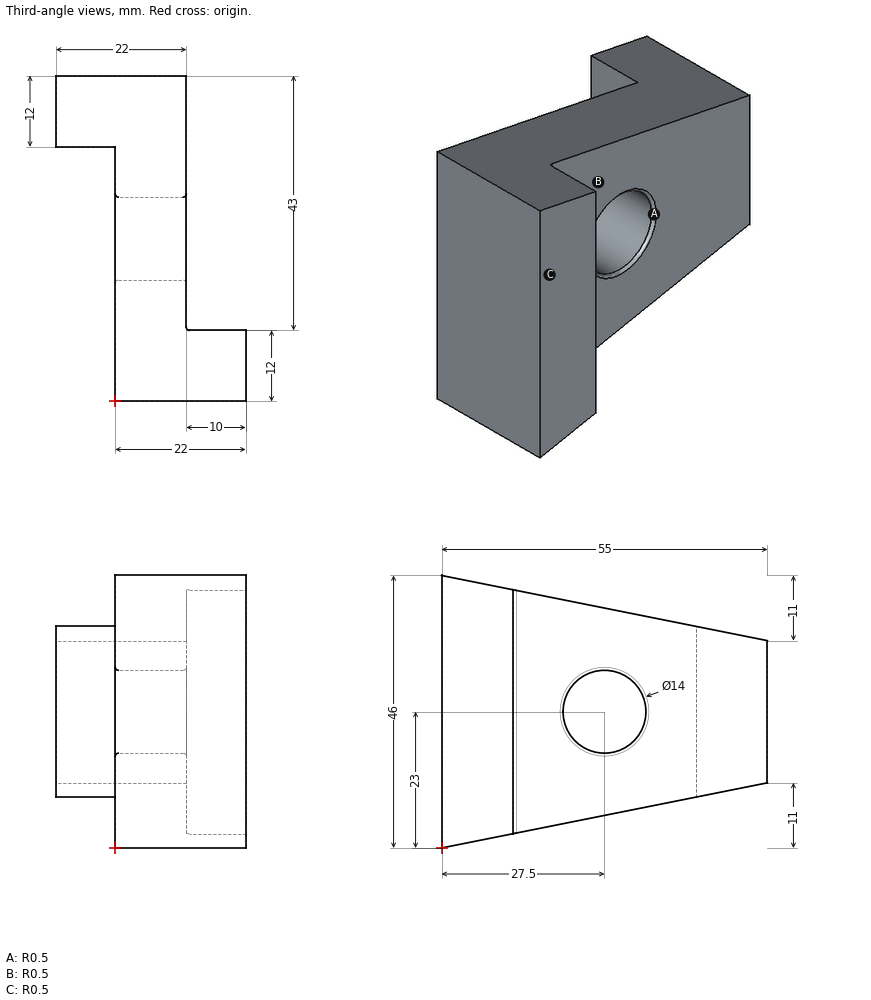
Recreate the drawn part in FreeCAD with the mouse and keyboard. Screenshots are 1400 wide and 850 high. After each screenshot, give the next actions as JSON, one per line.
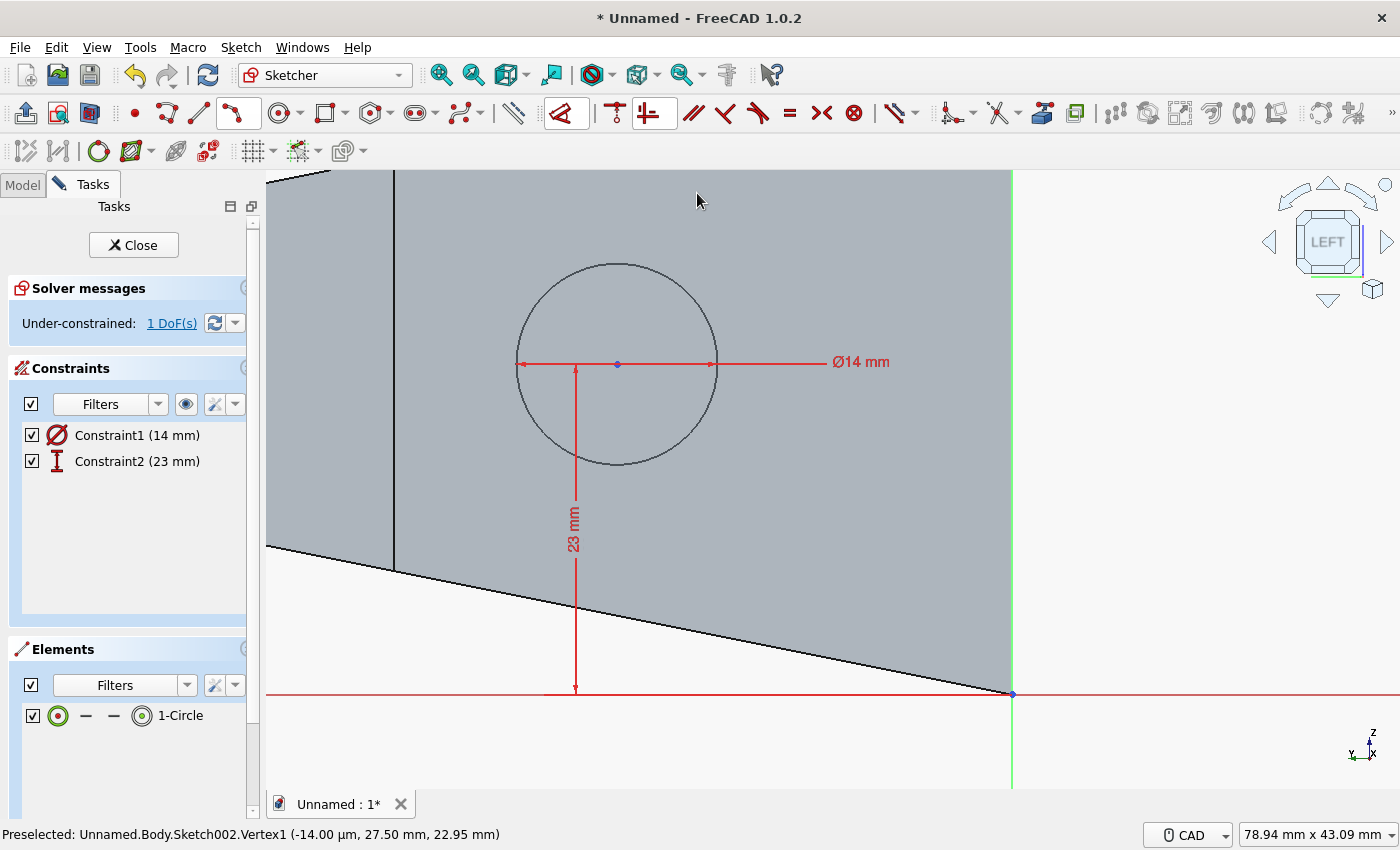
{"action": "left_click", "coordinate": [617, 364]}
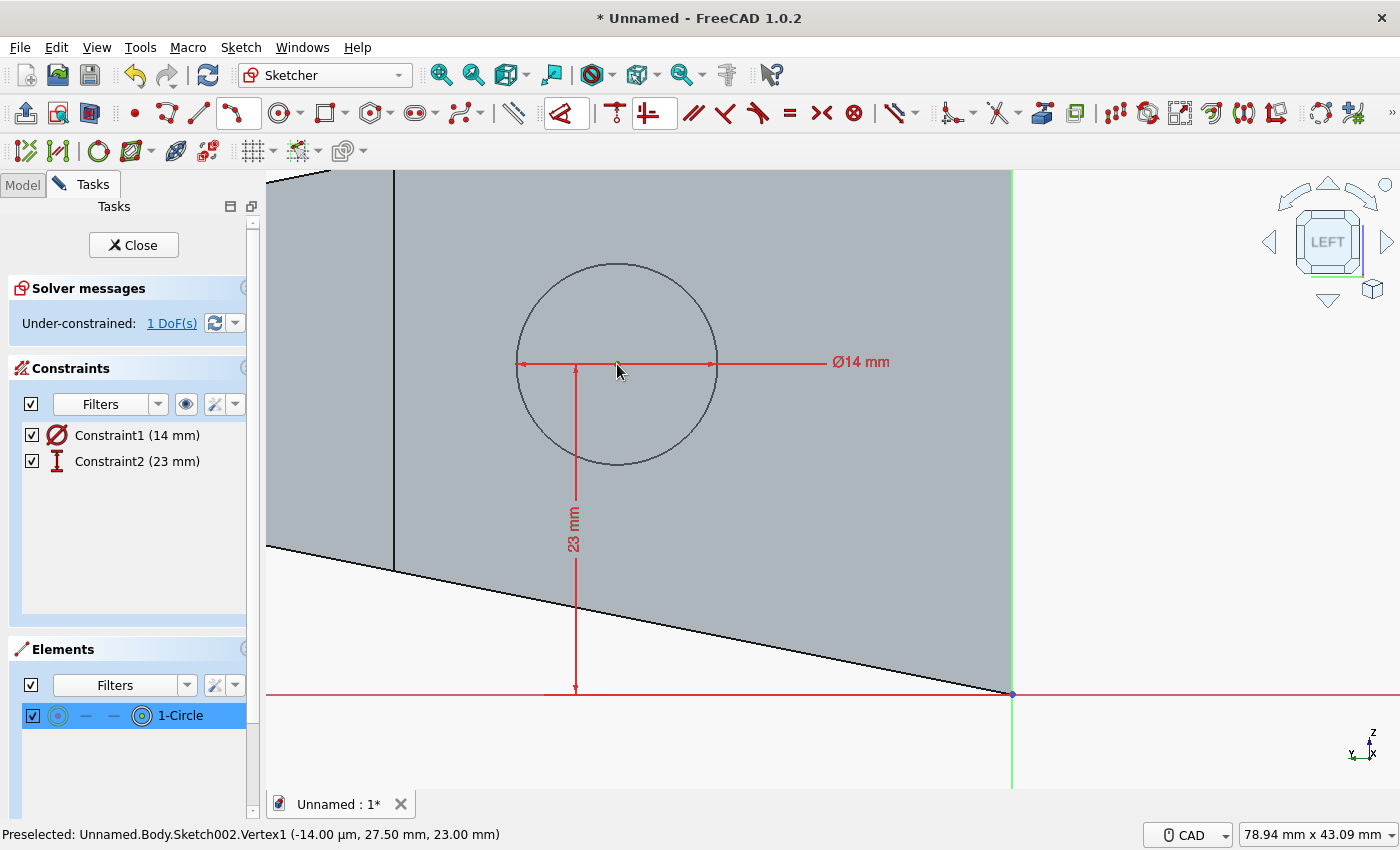
{"action": "left_click", "coordinate": [584, 114]}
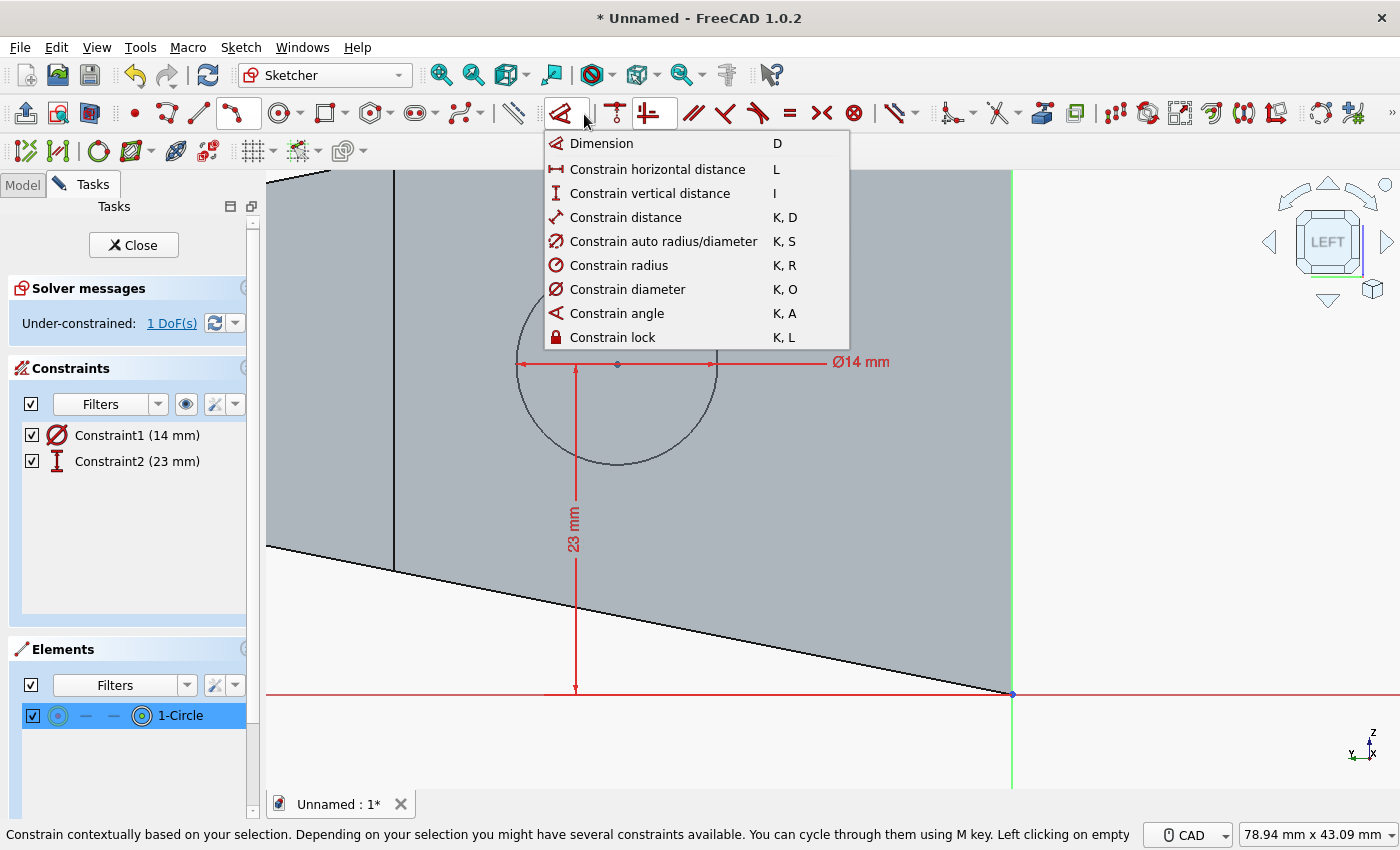
{"action": "left_click", "coordinate": [697, 169]}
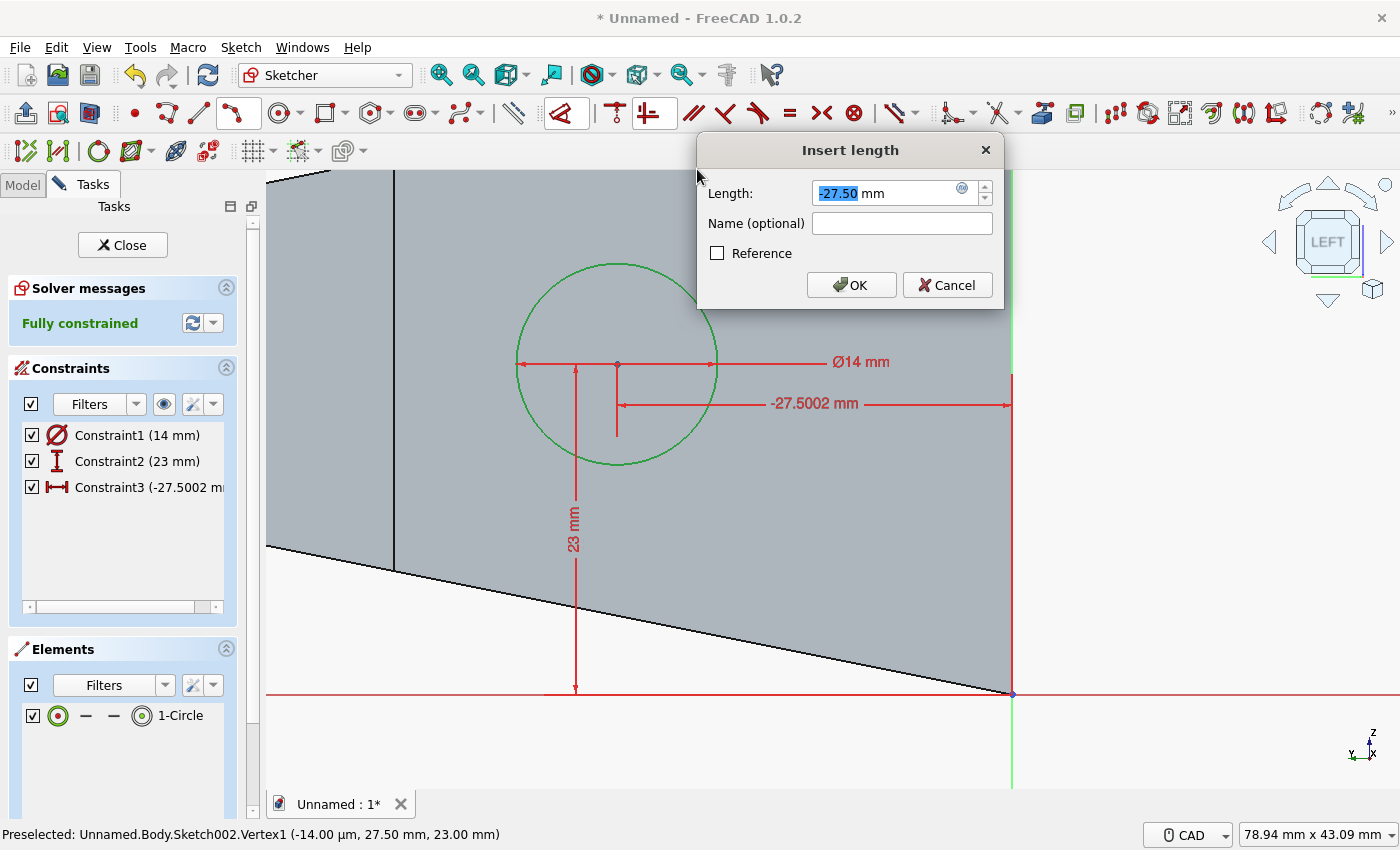
{"action": "type", "text": "-27.5"}
{"action": "key", "text": "Return"}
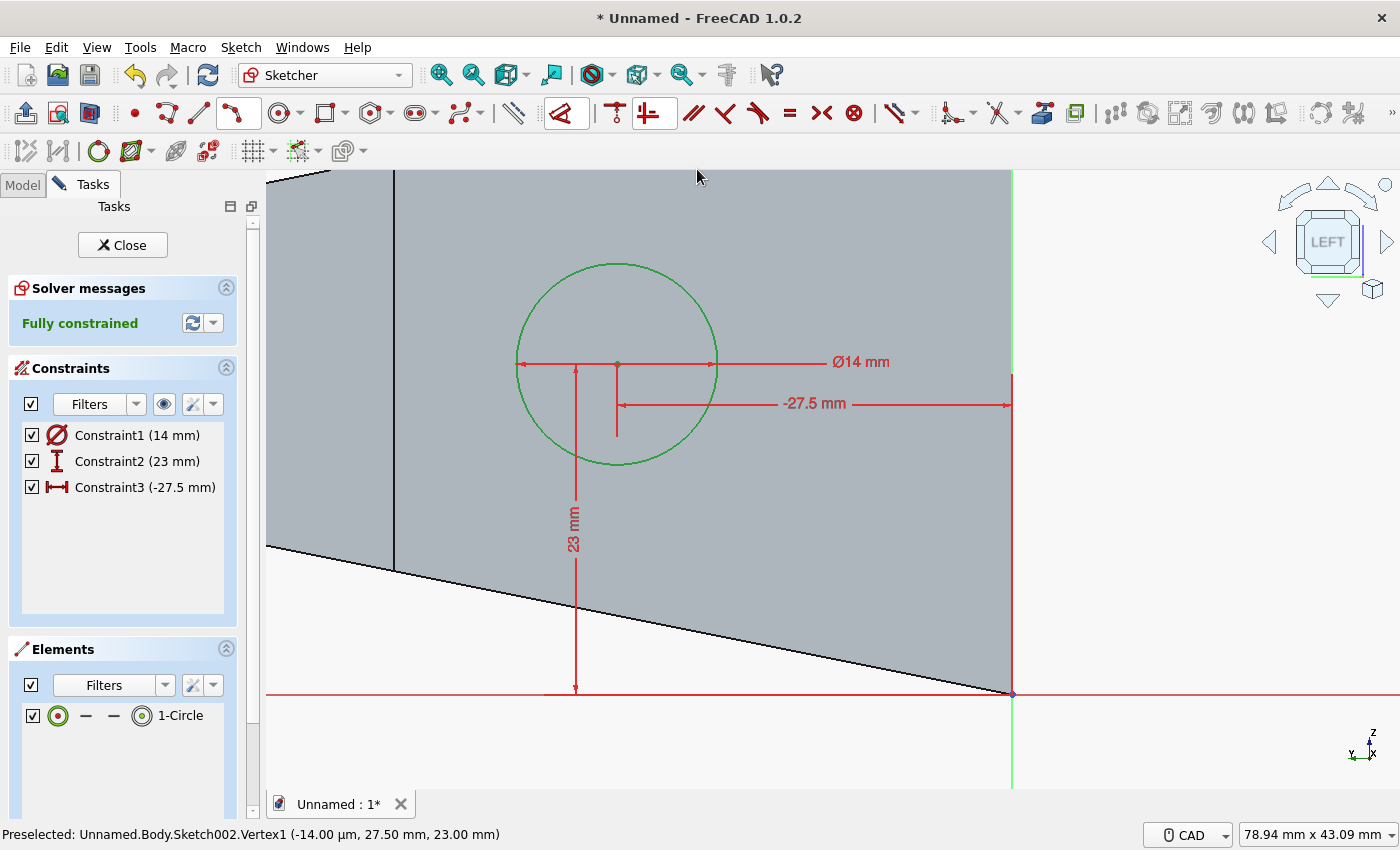
{"action": "left_click", "coordinate": [123, 245]}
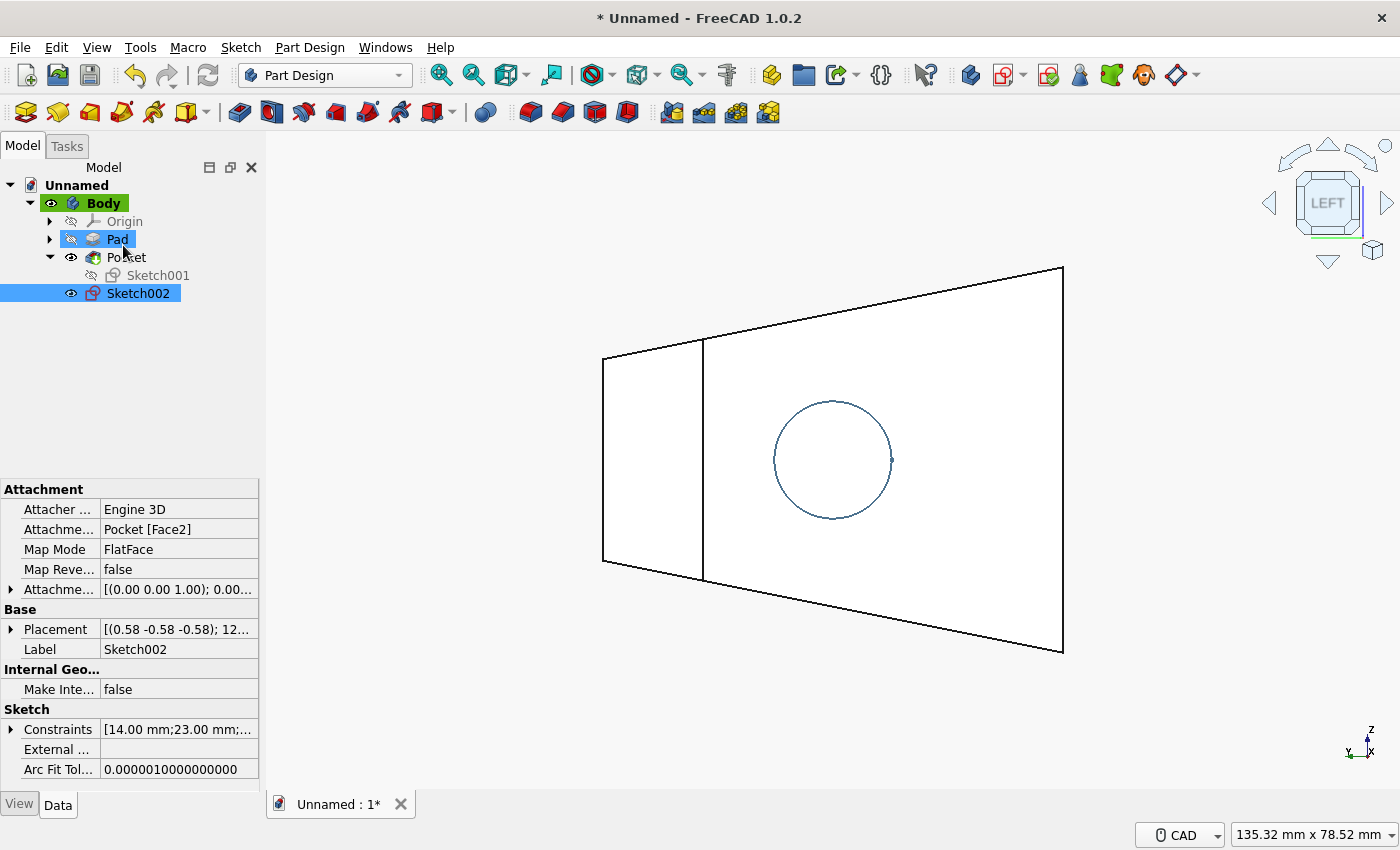
{"action": "left_click", "coordinate": [240, 112]}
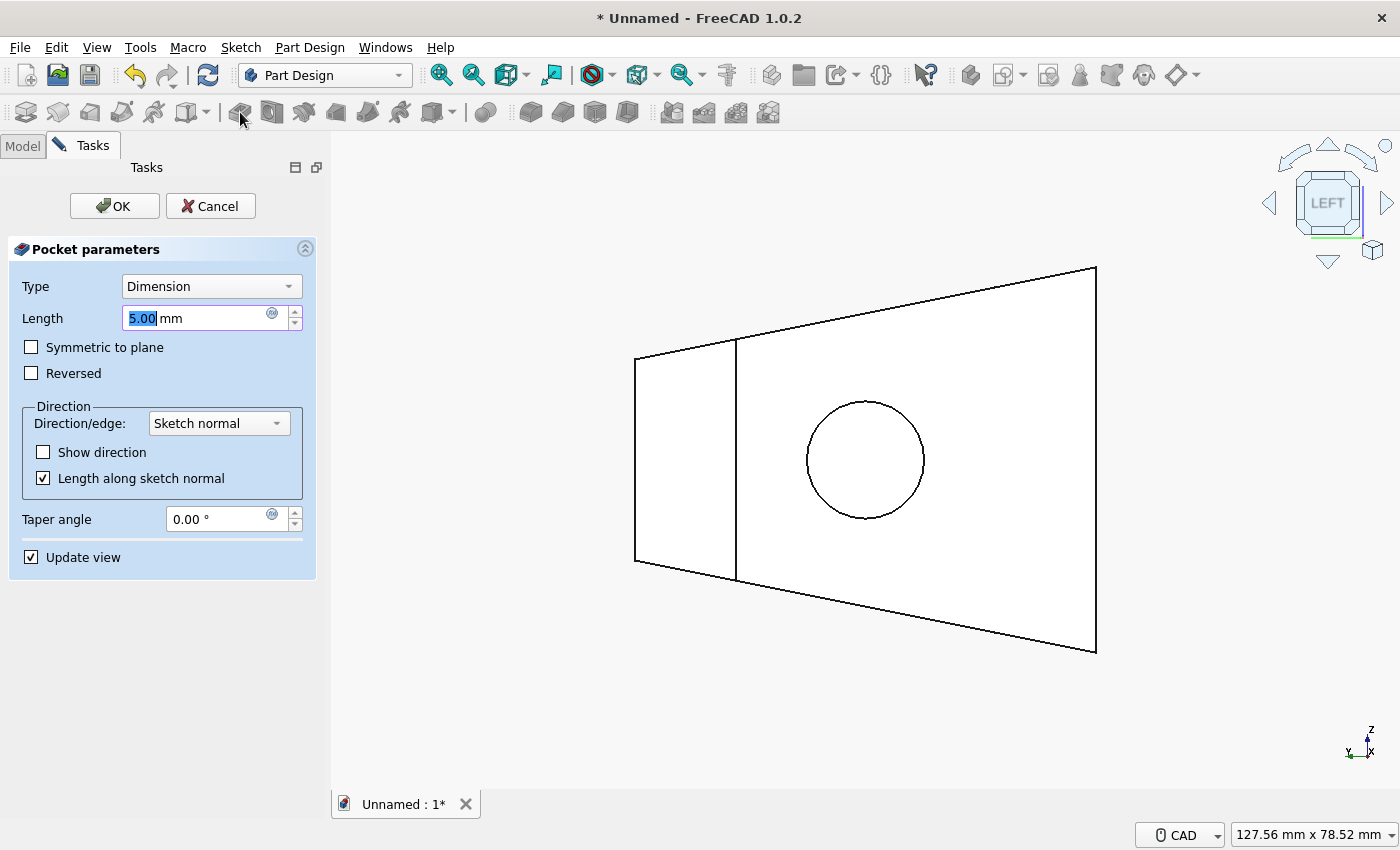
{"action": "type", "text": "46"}
{"action": "key", "text": "Tab"}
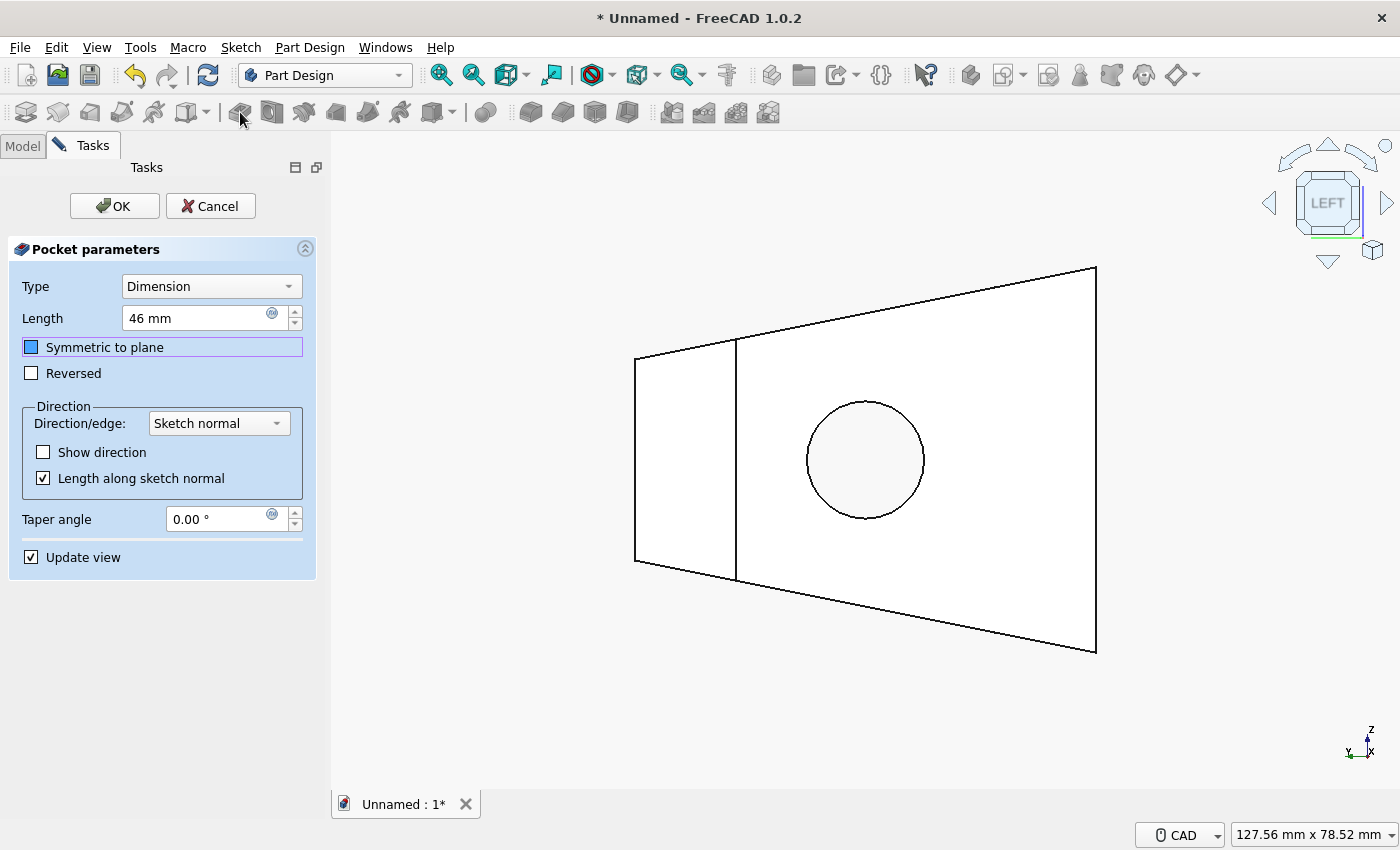
{"action": "left_click", "coordinate": [115, 206]}